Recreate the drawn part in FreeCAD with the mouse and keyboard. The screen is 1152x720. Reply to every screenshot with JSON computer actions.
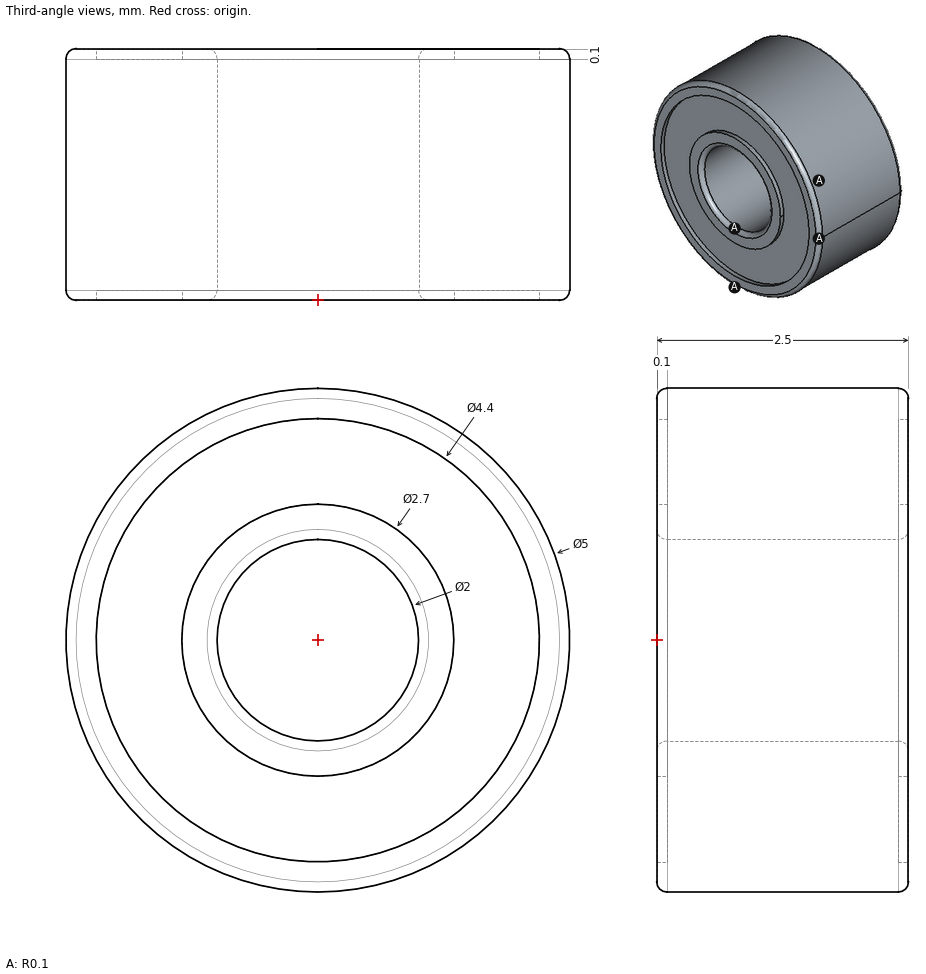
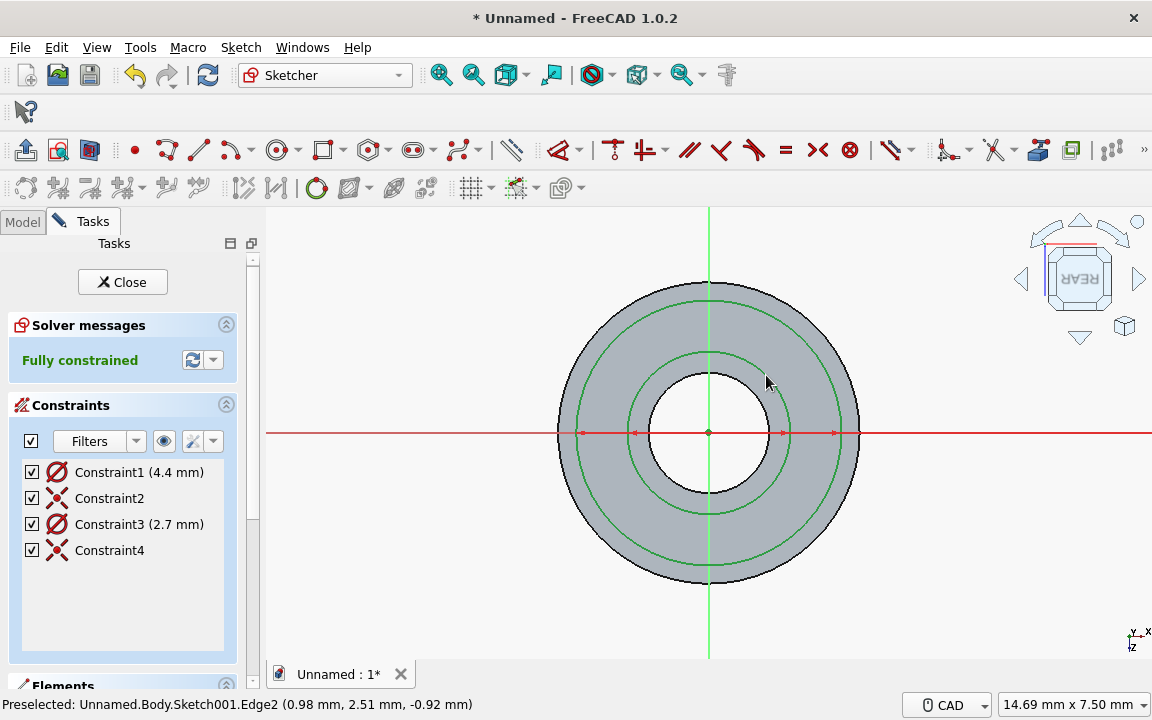
{"action": "left_click", "coordinate": [123, 282]}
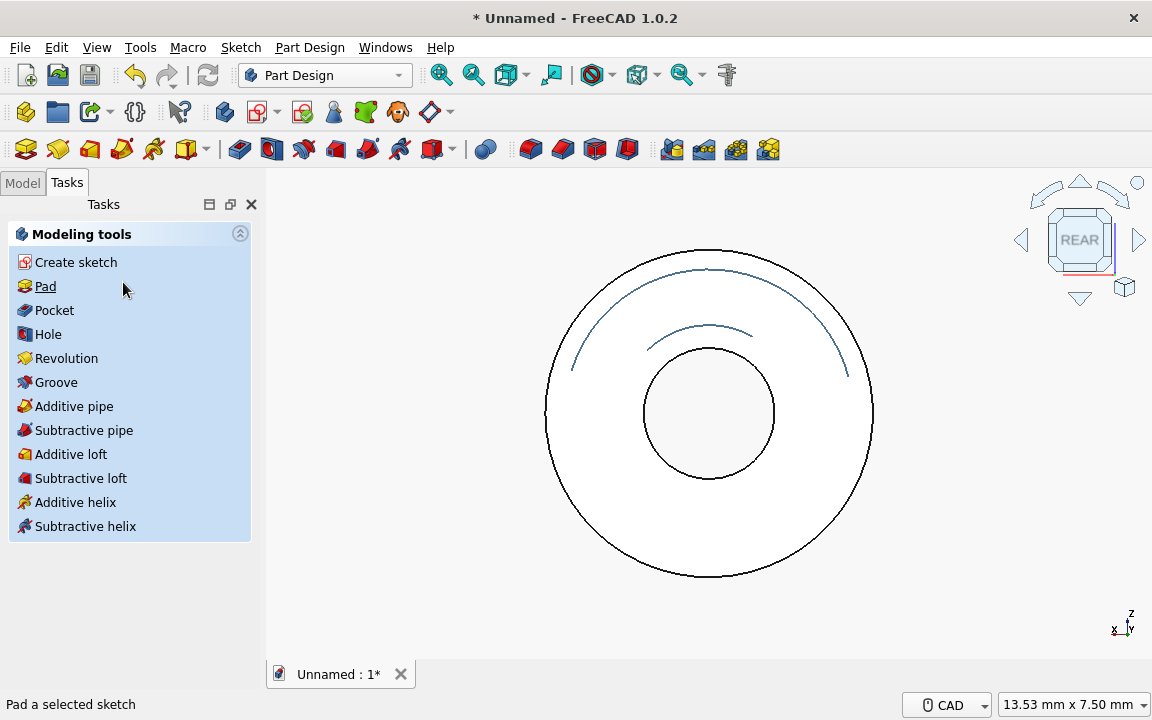
{"action": "left_click", "coordinate": [240, 150]}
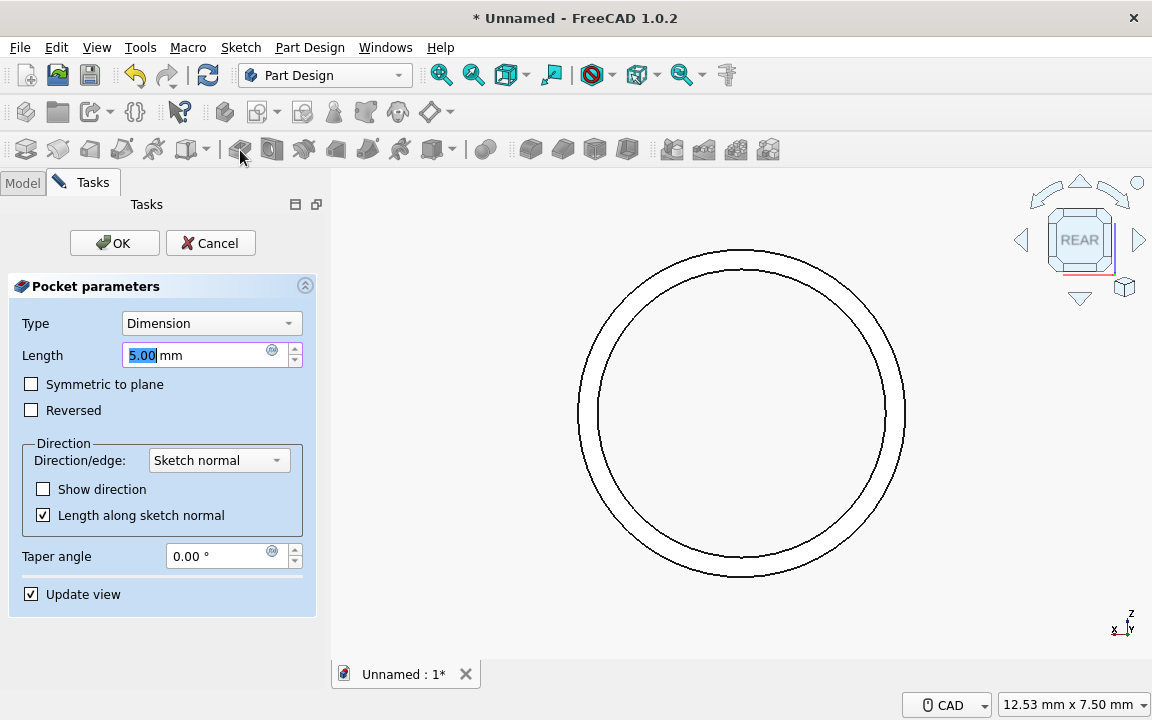
{"action": "type", "text": "0.1"}
{"action": "key", "text": "Tab"}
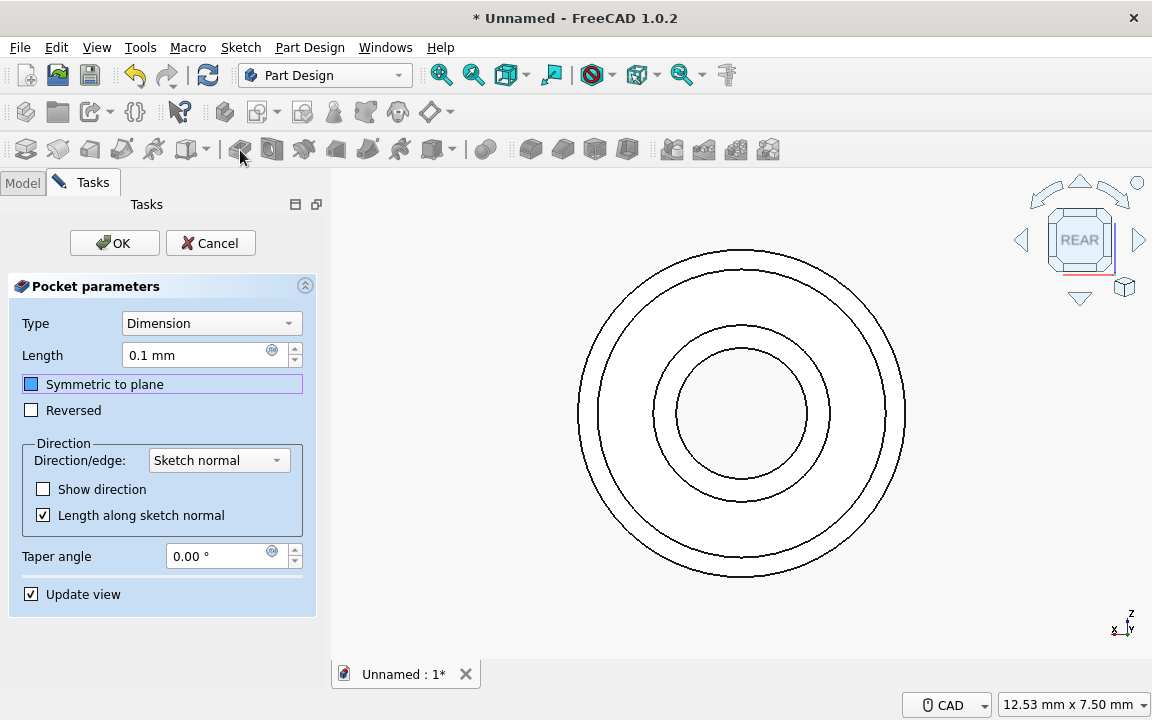
{"action": "left_click", "coordinate": [115, 243]}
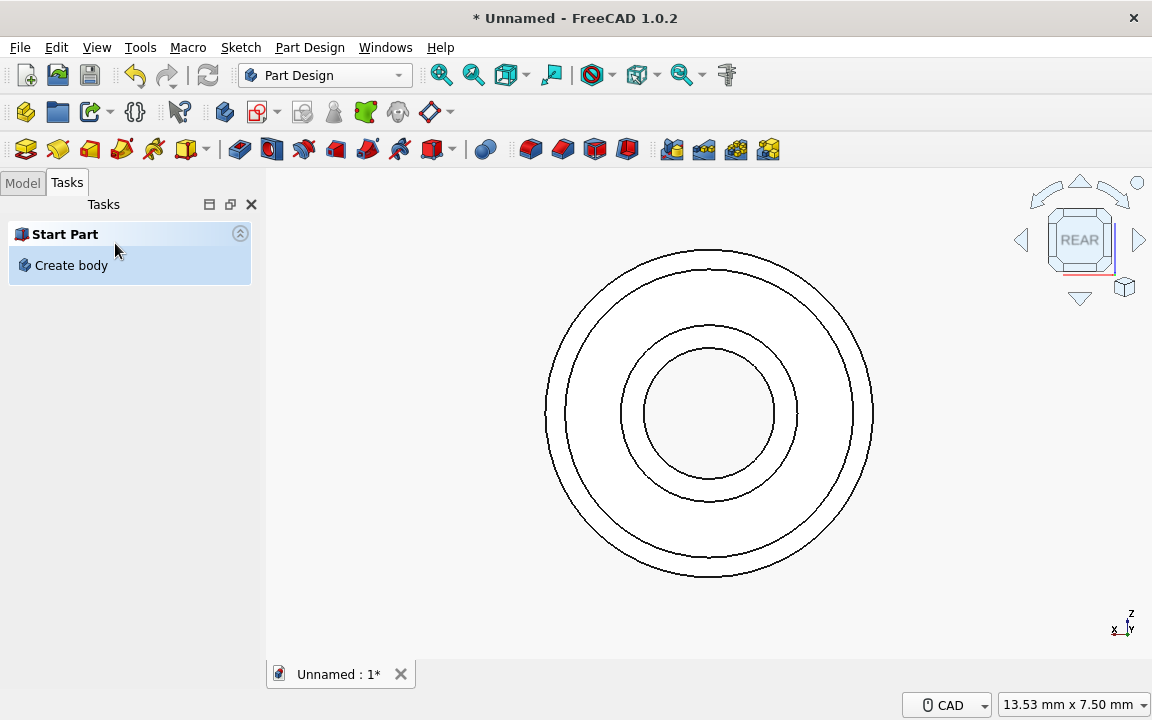
{"action": "left_click", "coordinate": [23, 182]}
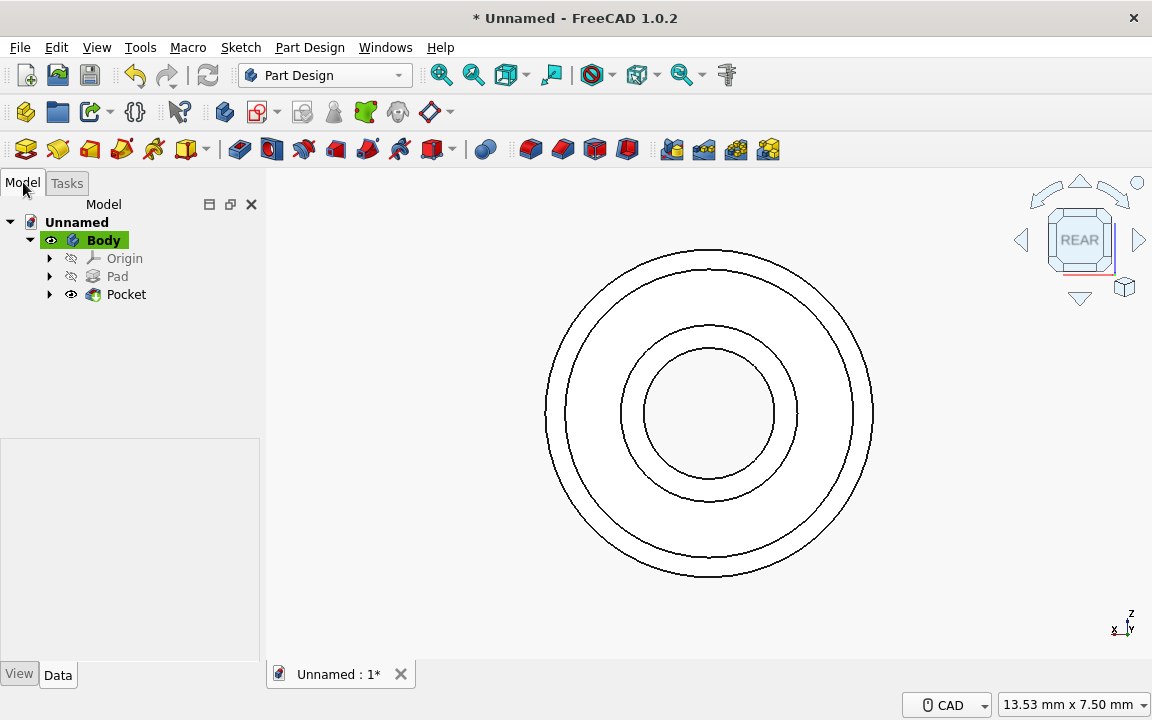
{"action": "left_click", "coordinate": [50, 258]}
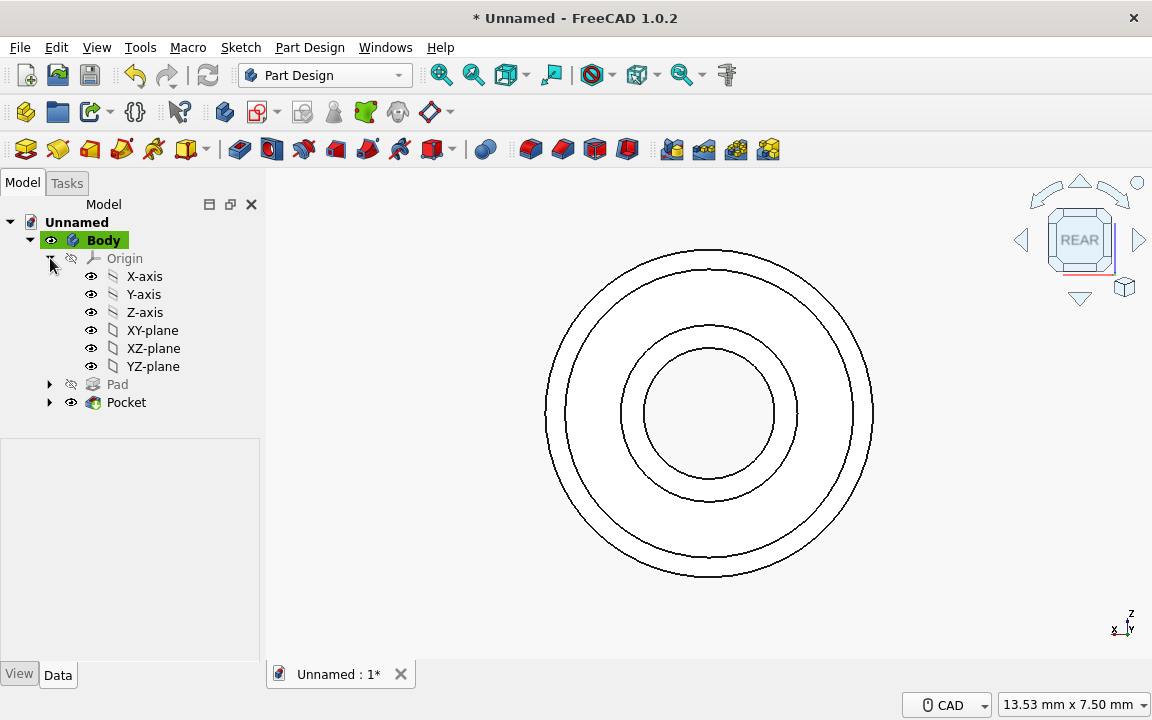
{"action": "left_click", "coordinate": [136, 348]}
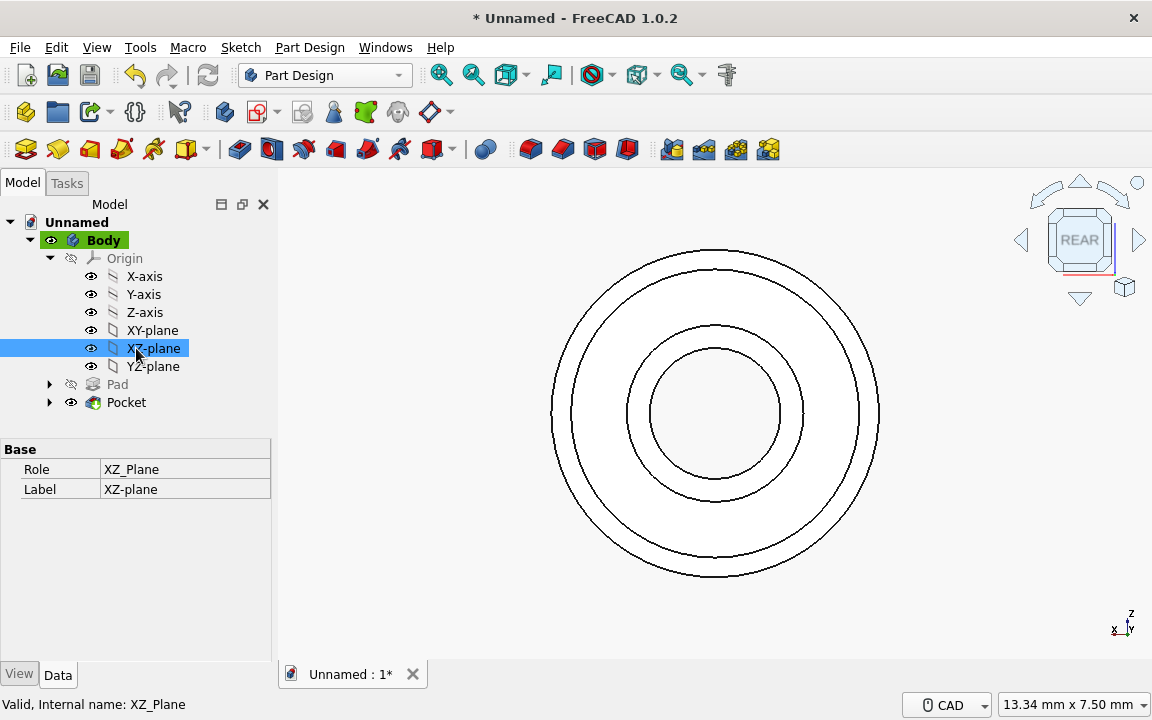
{"action": "left_click", "coordinate": [430, 112]}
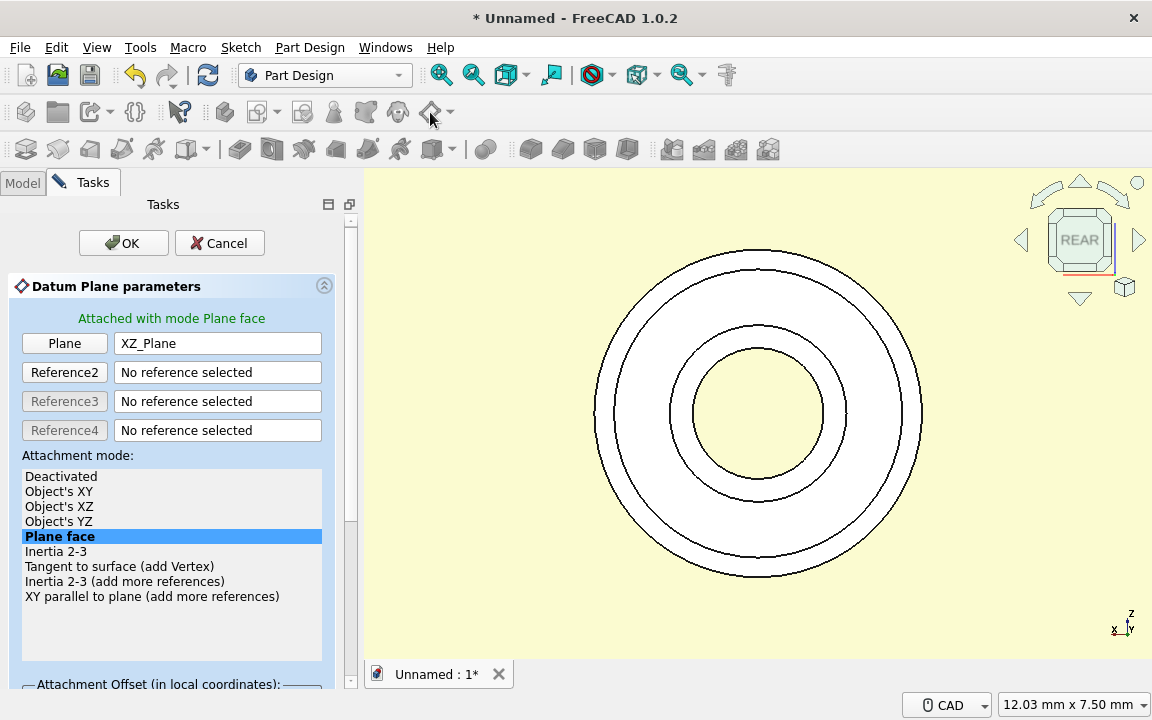
{"action": "scroll", "coordinate": [351, 451], "scroll_direction": "down", "scroll_amount": 3}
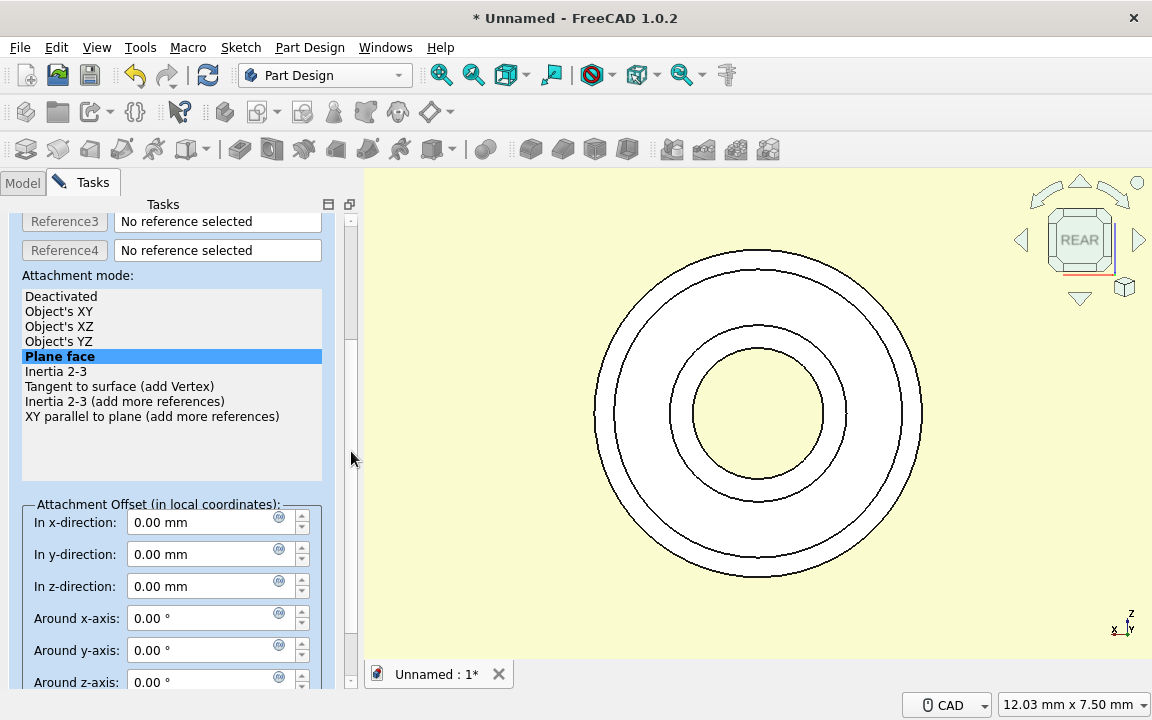
{"action": "triple_click", "coordinate": [210, 586]}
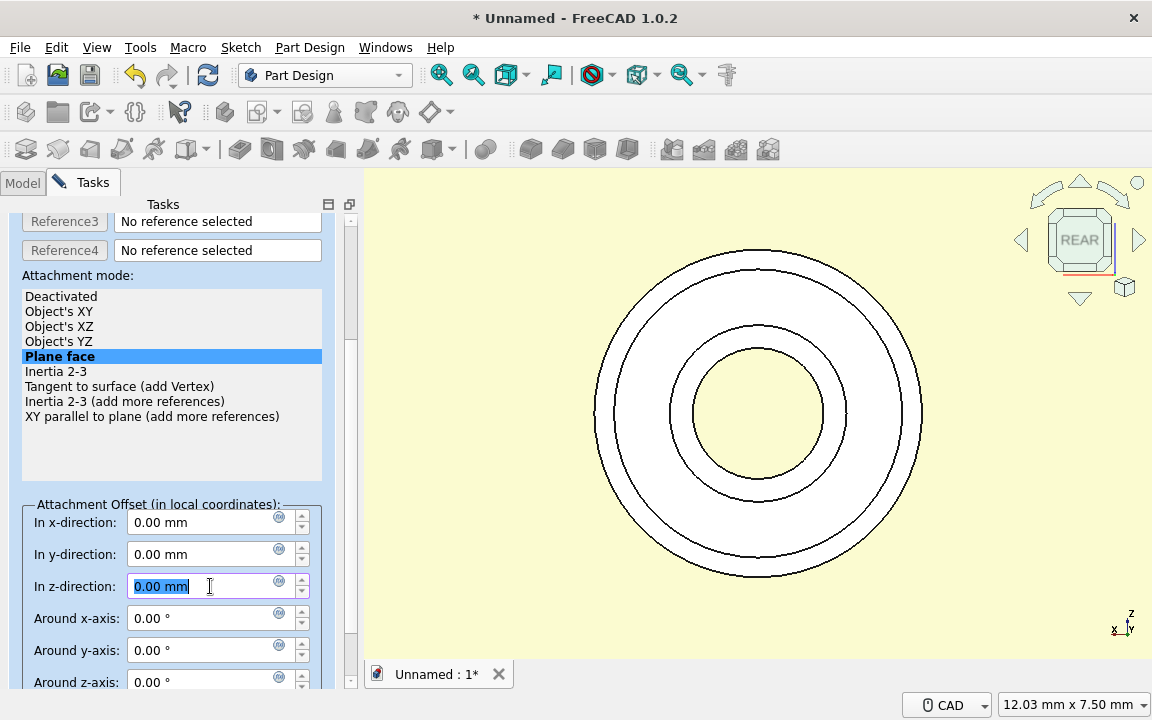
{"action": "type", "text": "-0.1"}
{"action": "key", "text": "Tab"}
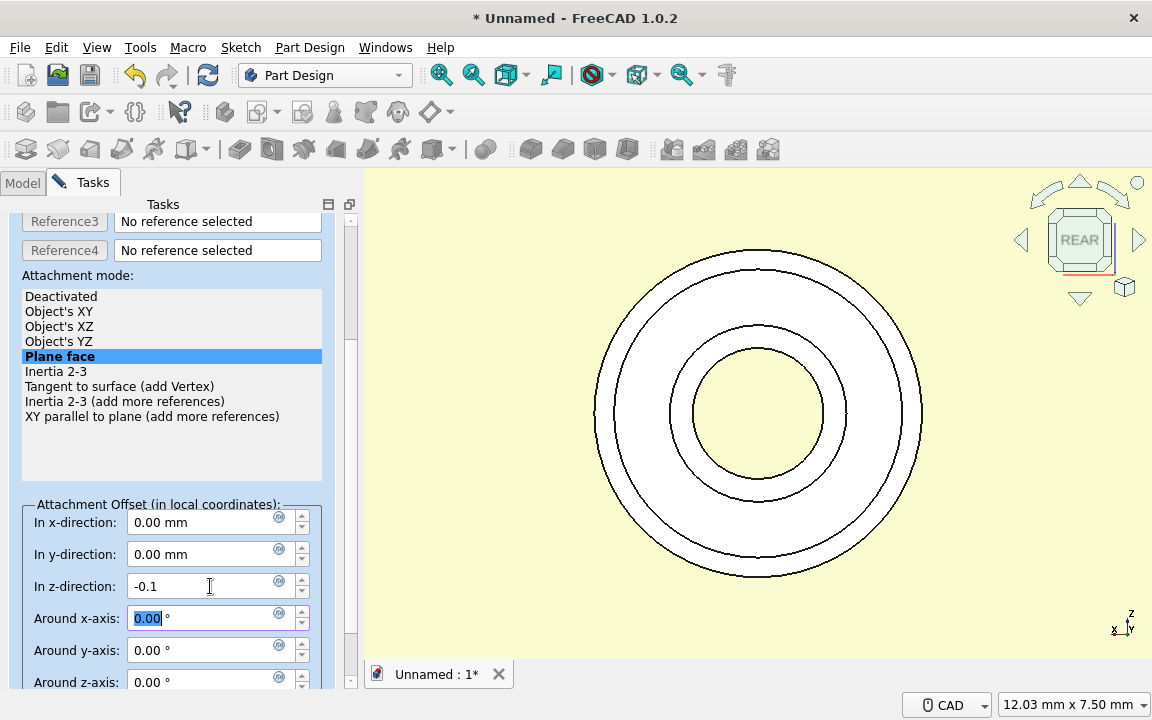
{"action": "scroll", "coordinate": [351, 451], "scroll_direction": "up", "scroll_amount": 4}